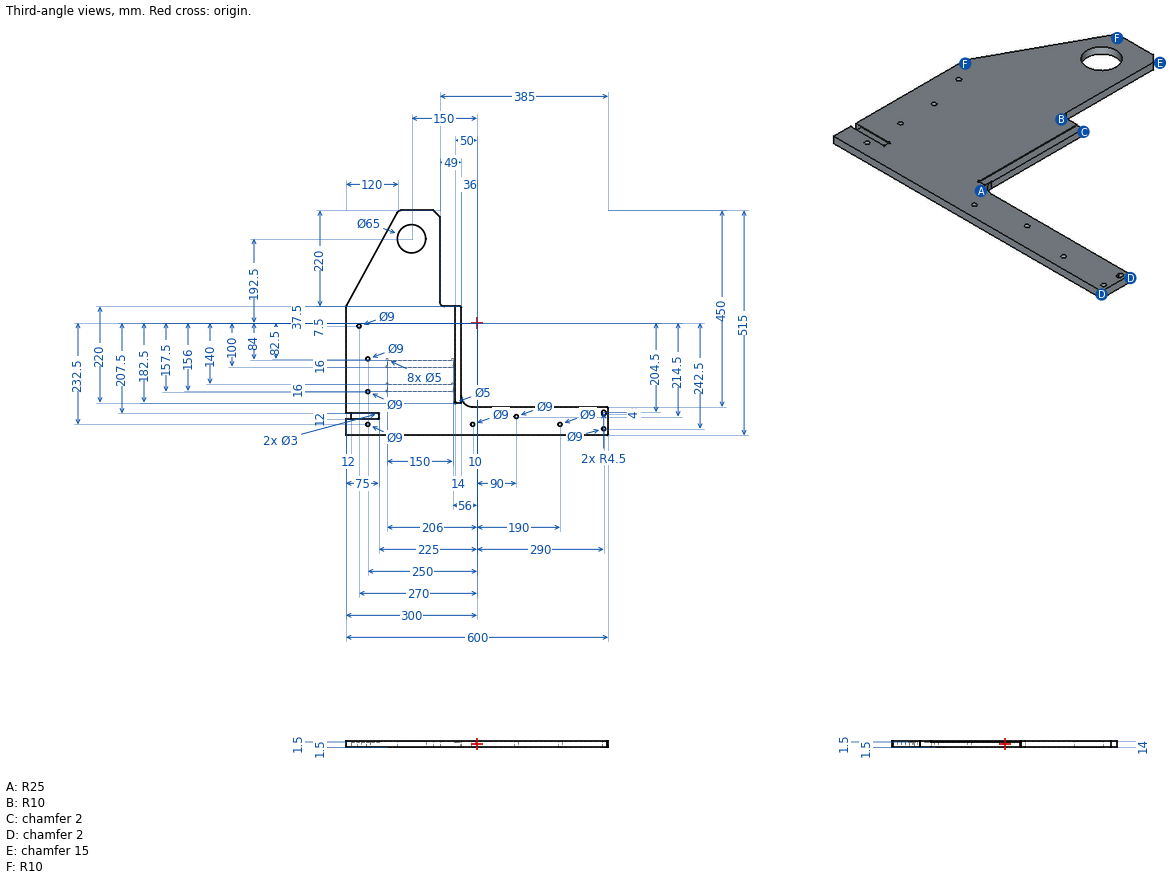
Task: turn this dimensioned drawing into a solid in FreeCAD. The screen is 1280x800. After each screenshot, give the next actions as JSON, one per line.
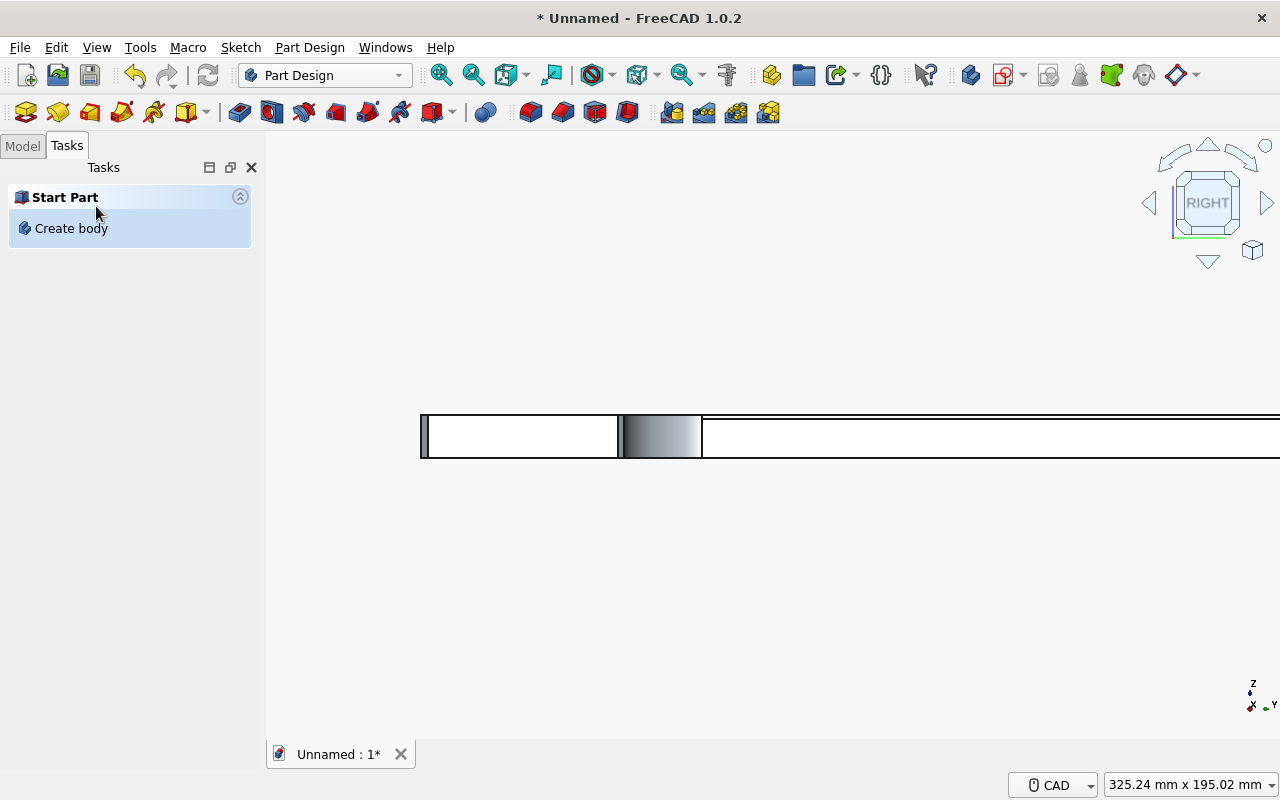
{"action": "left_click", "coordinate": [442, 76]}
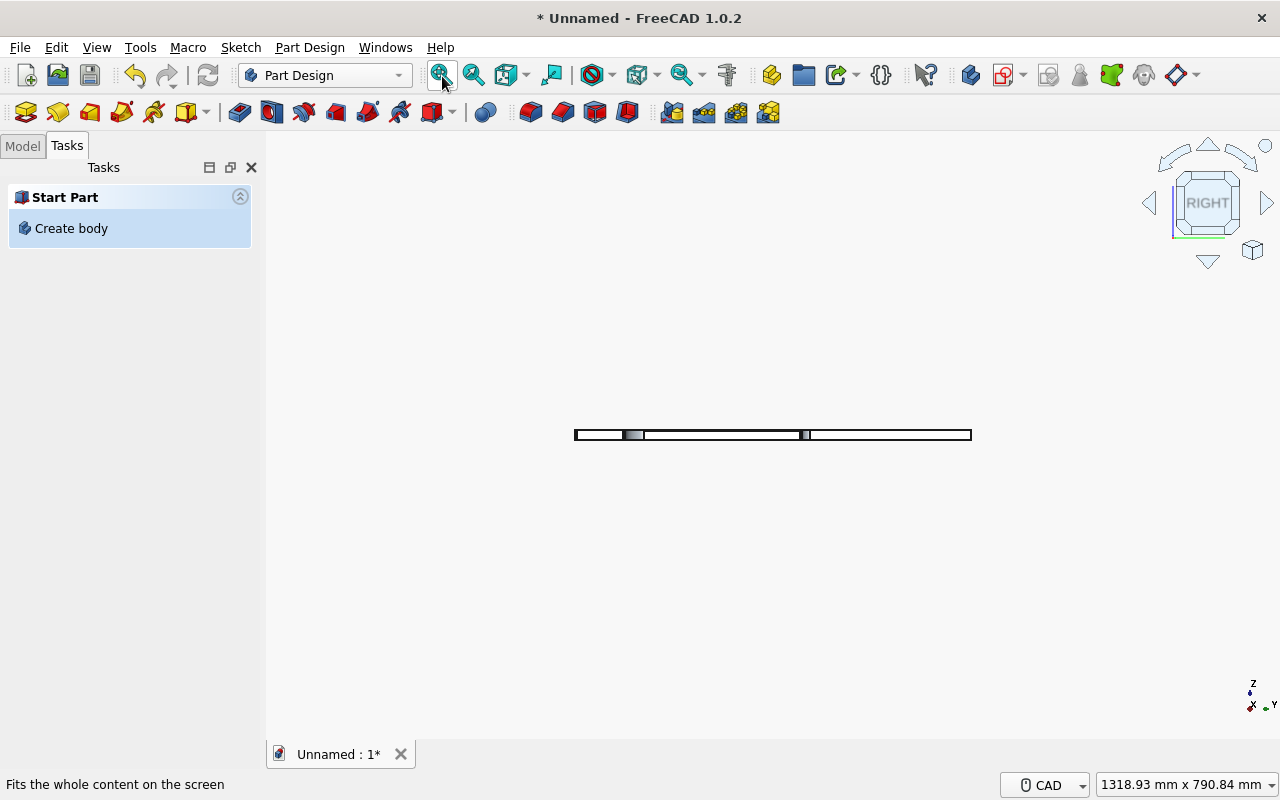
{"action": "key", "text": "0"}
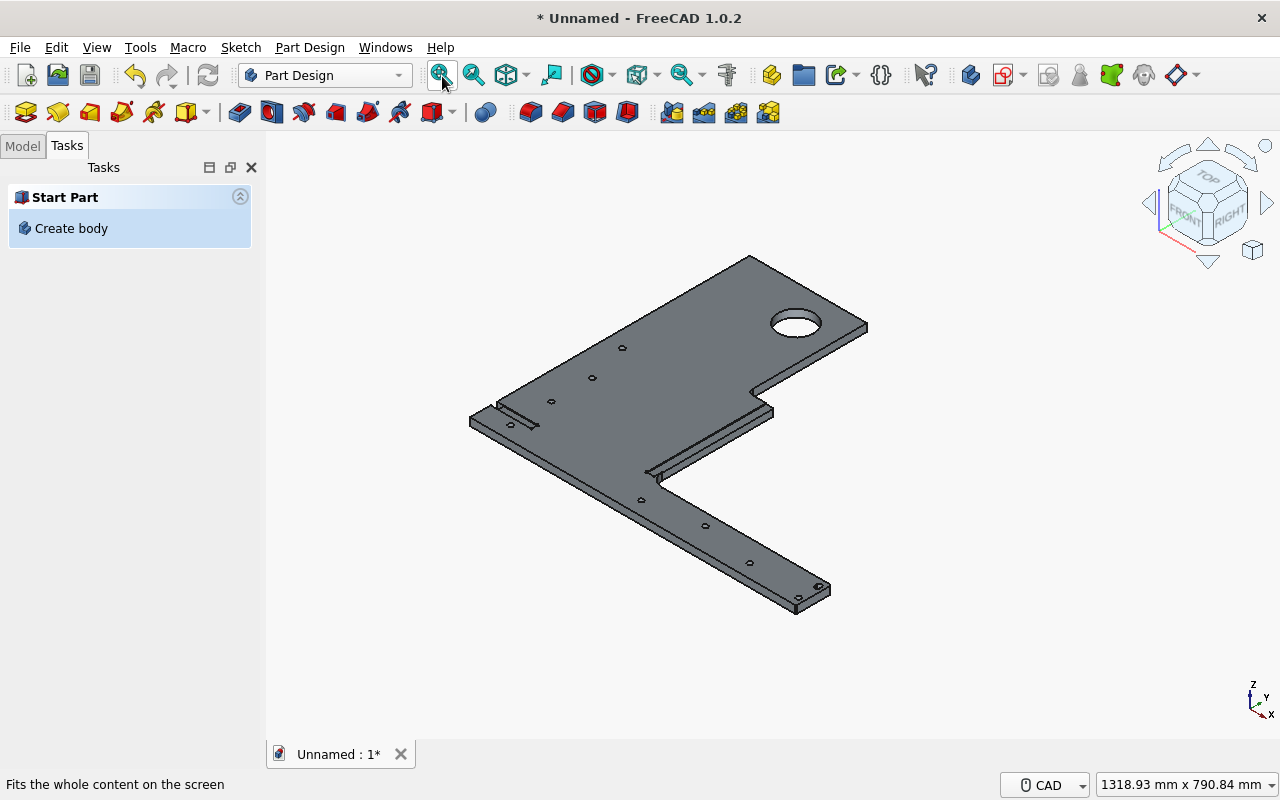
{"action": "left_click", "coordinate": [680, 376]}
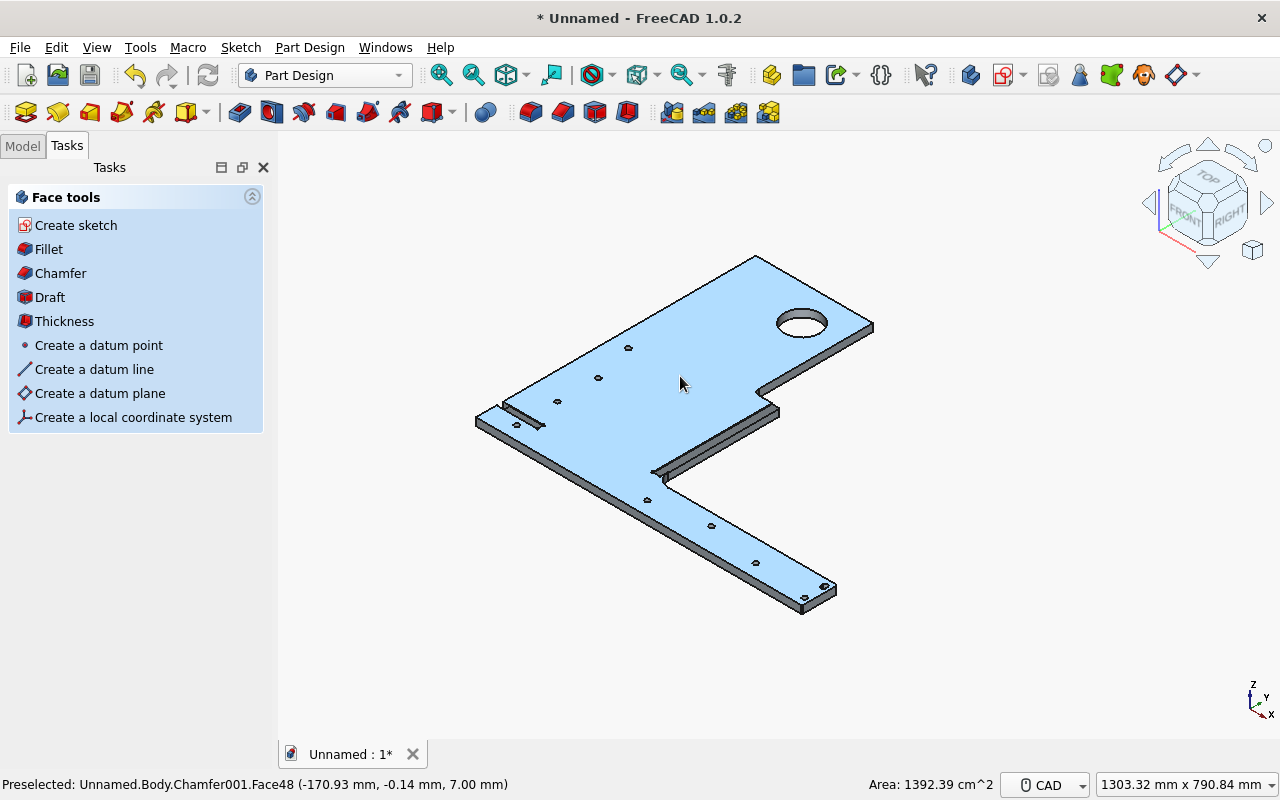
{"action": "left_click", "coordinate": [1004, 76]}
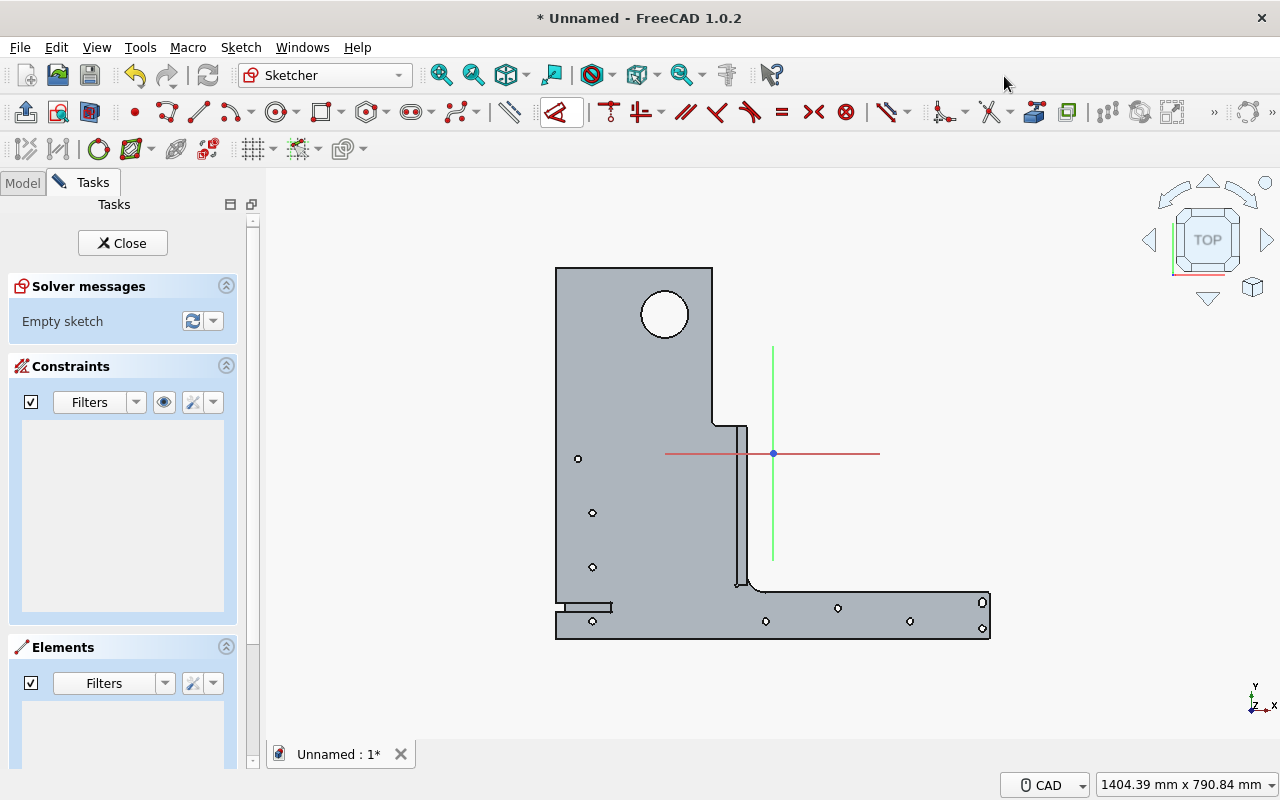
{"action": "scroll", "coordinate": [616, 247], "scroll_direction": "up", "scroll_amount": 3}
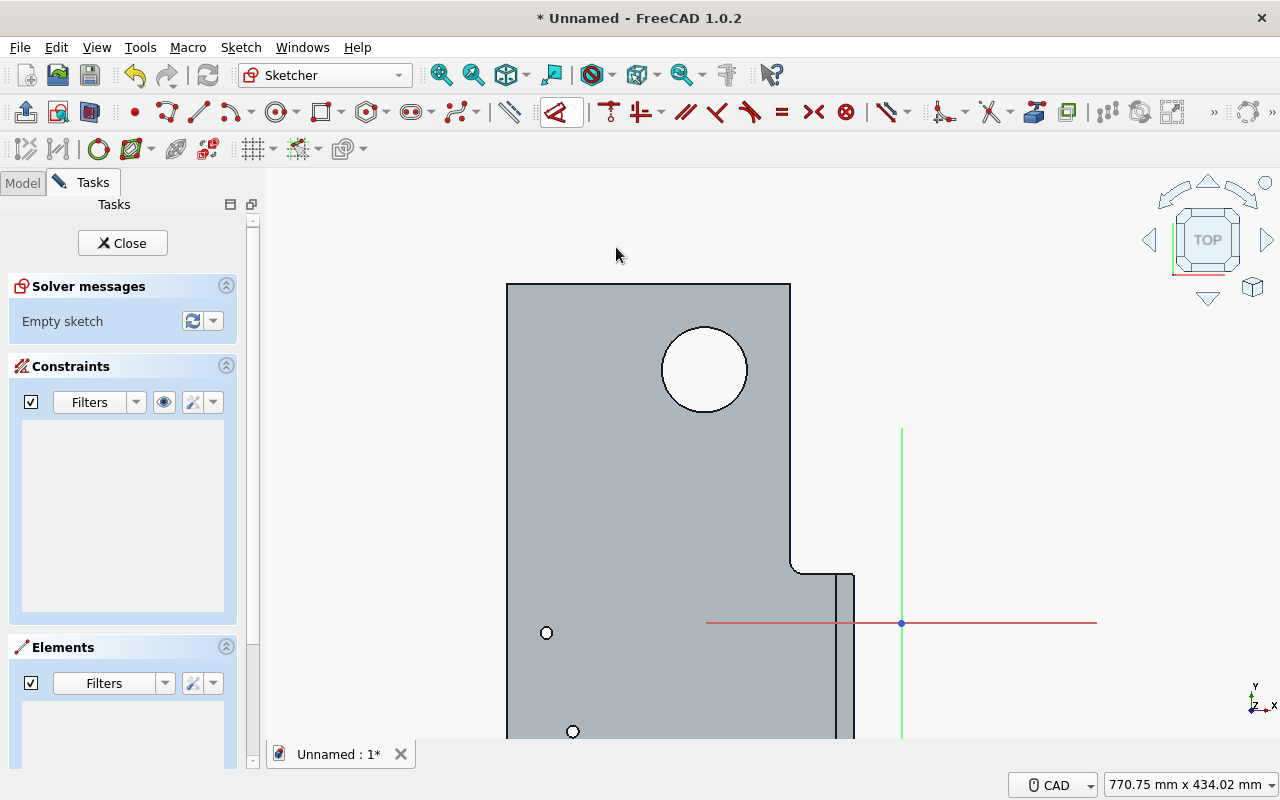
{"action": "left_click", "coordinate": [168, 112]}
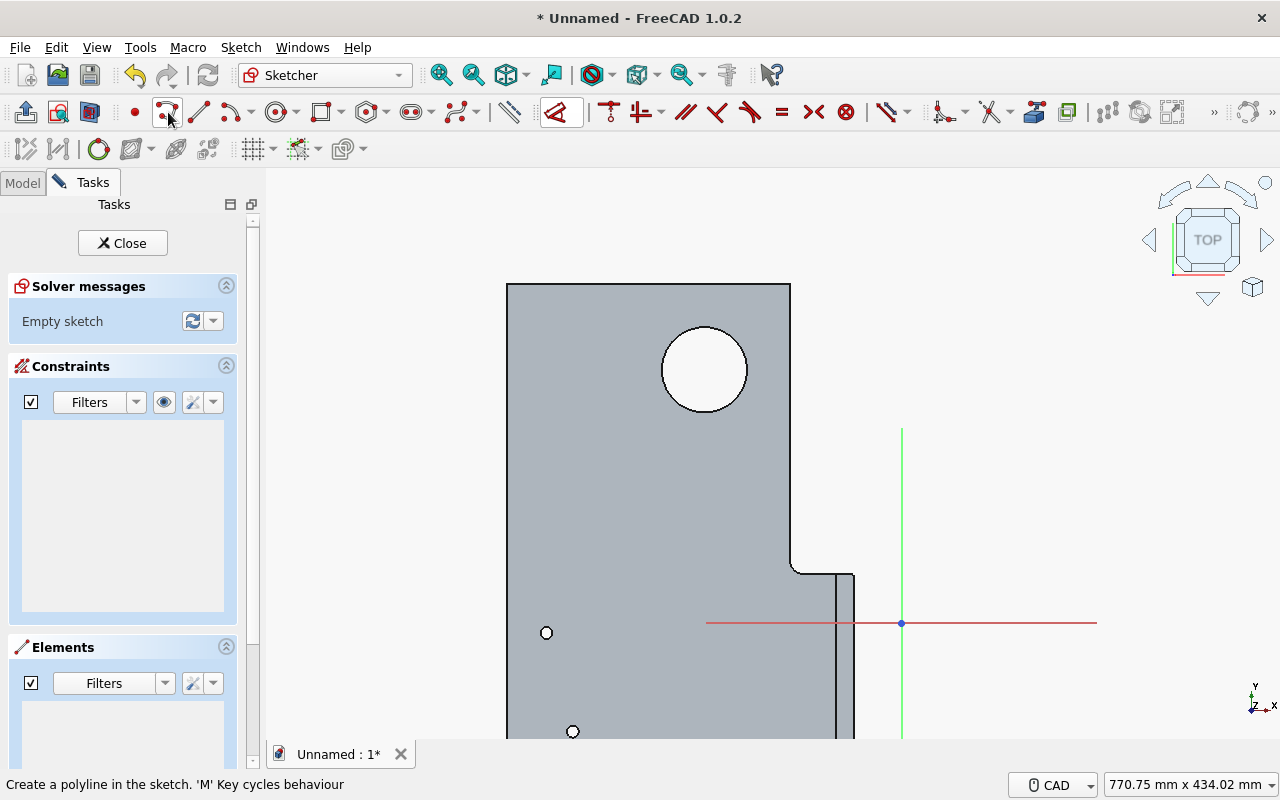
{"action": "left_click", "coordinate": [507, 574]}
{"action": "left_click", "coordinate": [665, 284]}
{"action": "left_click", "coordinate": [507, 284]}
{"action": "left_click", "coordinate": [507, 575]}
{"action": "key", "text": "Escape"}
{"action": "key", "text": "Escape"}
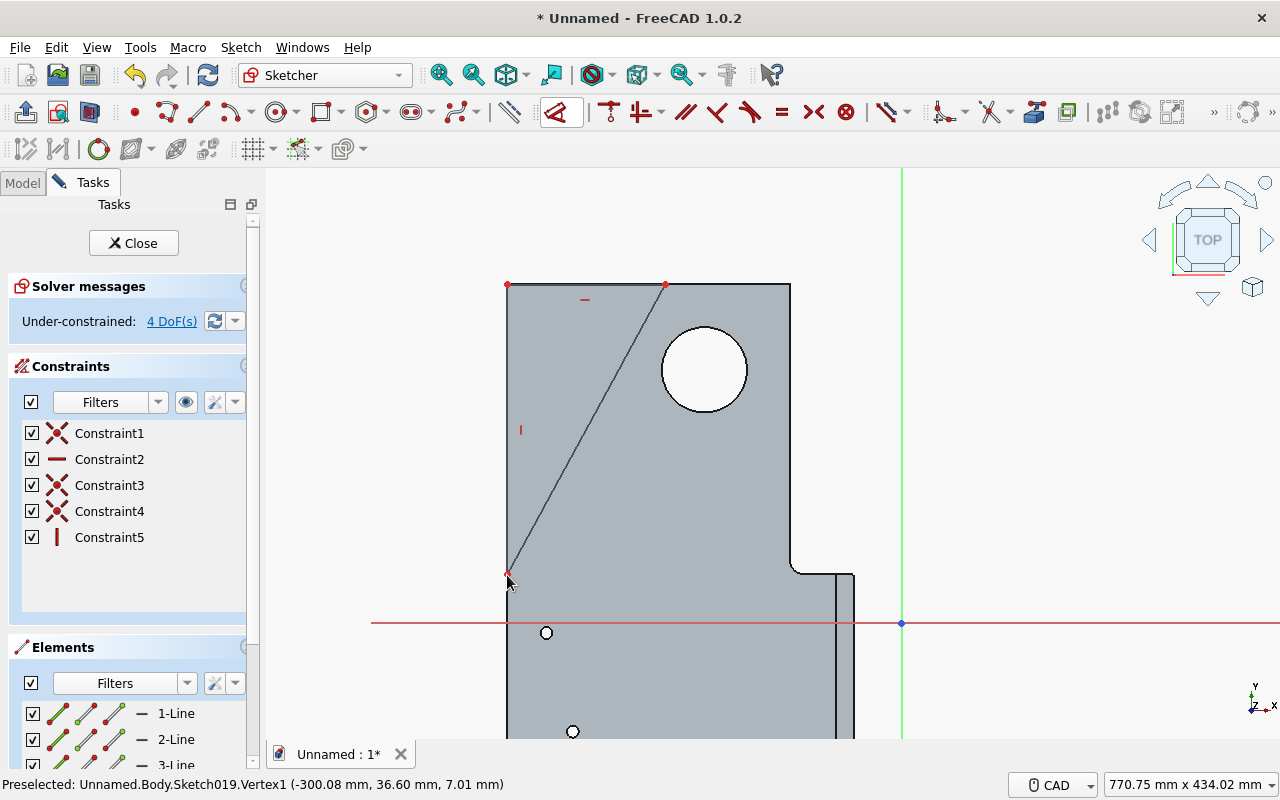
{"action": "left_click", "coordinate": [618, 285]}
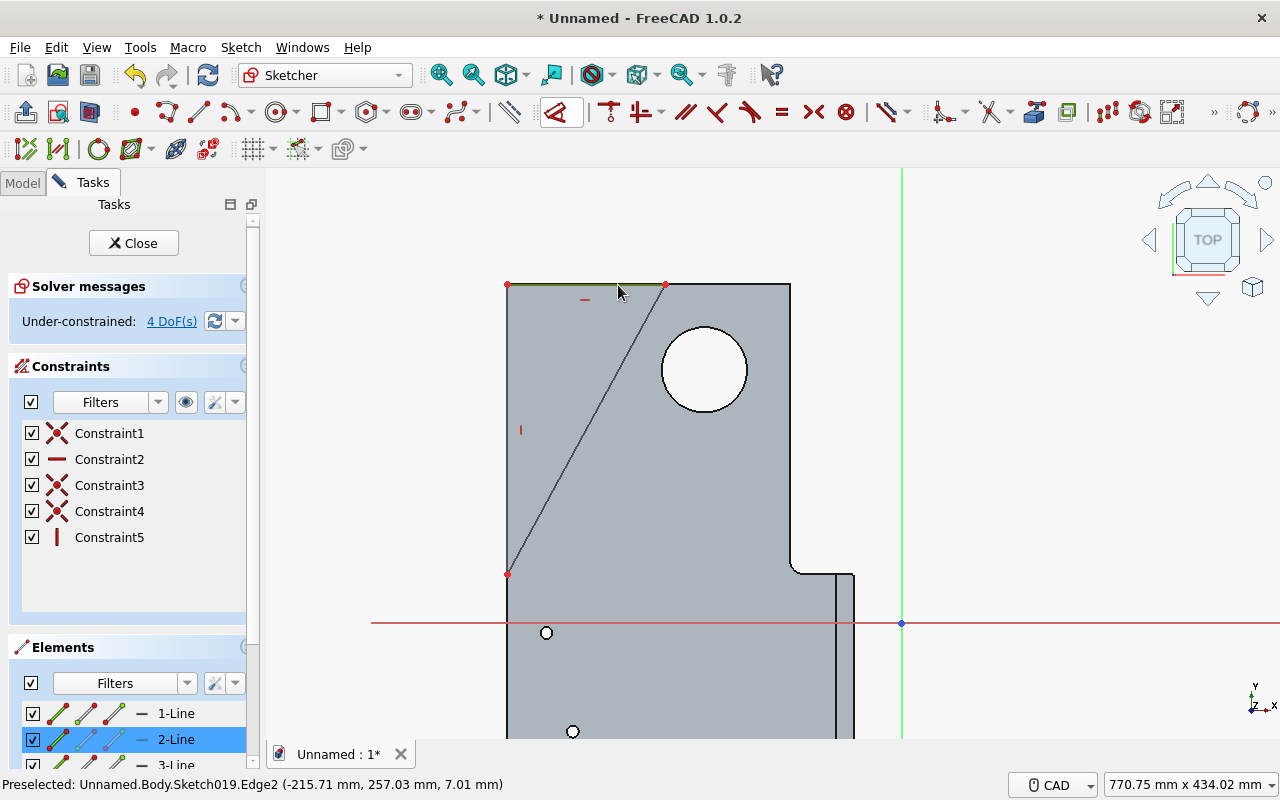
{"action": "left_click", "coordinate": [578, 112]}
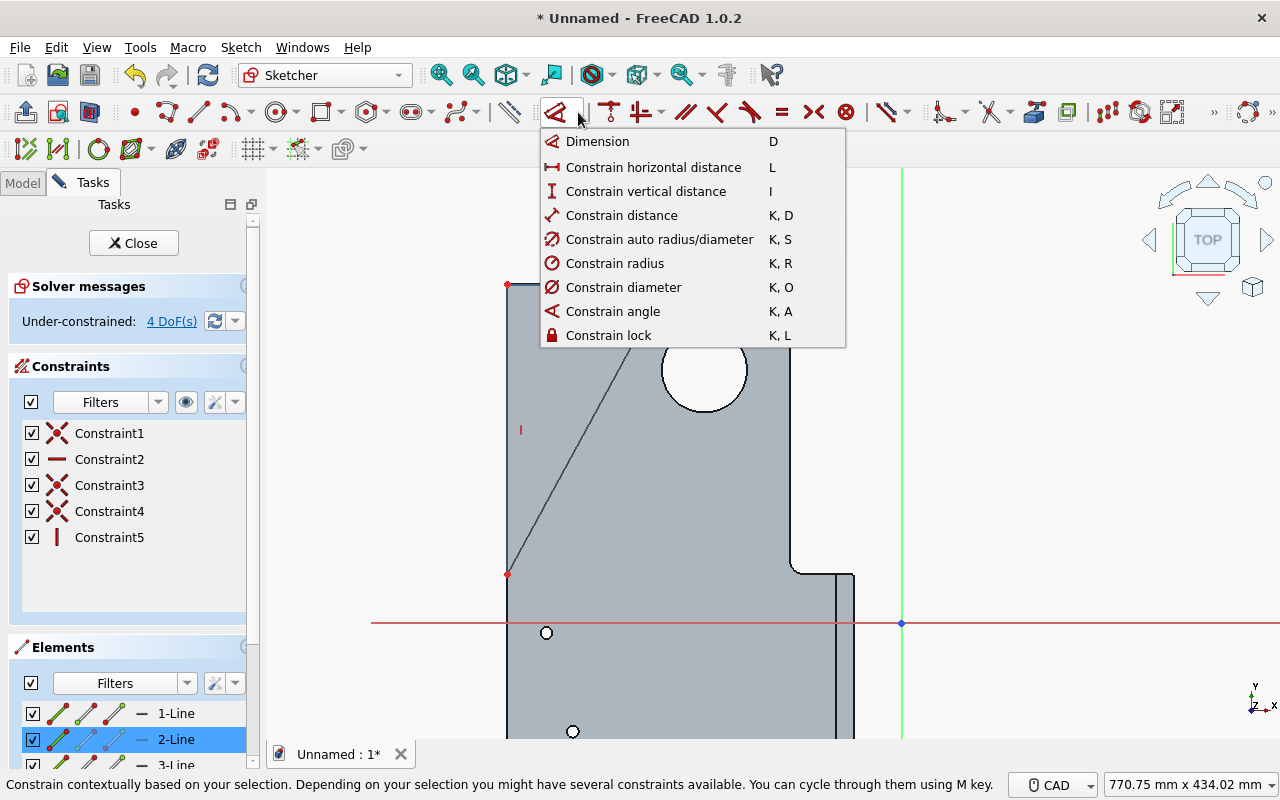
{"action": "left_click", "coordinate": [693, 167]}